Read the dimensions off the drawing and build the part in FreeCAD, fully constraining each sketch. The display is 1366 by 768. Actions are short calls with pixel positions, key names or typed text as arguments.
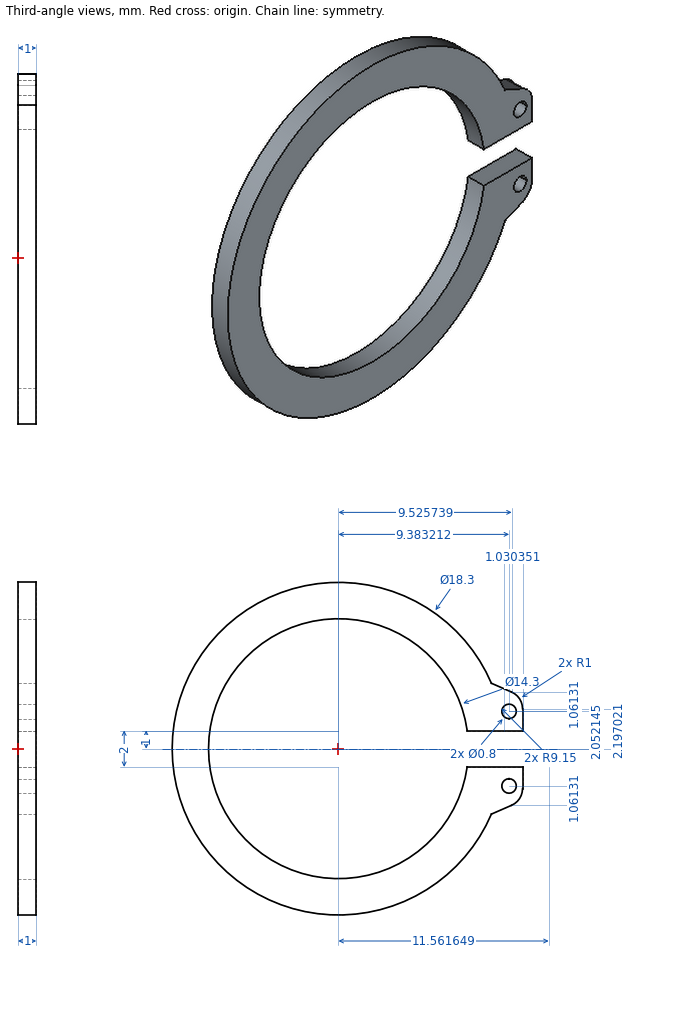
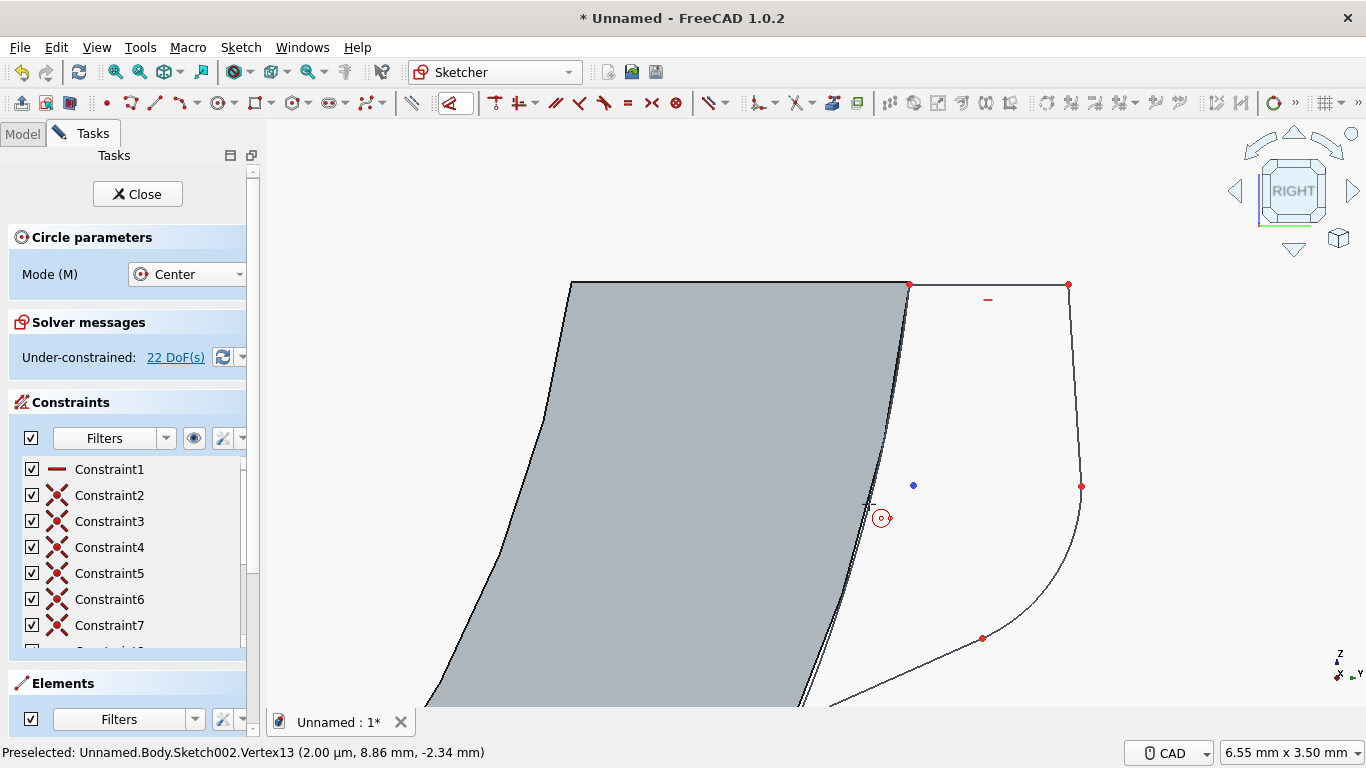
scroll(969, 542, down, 6)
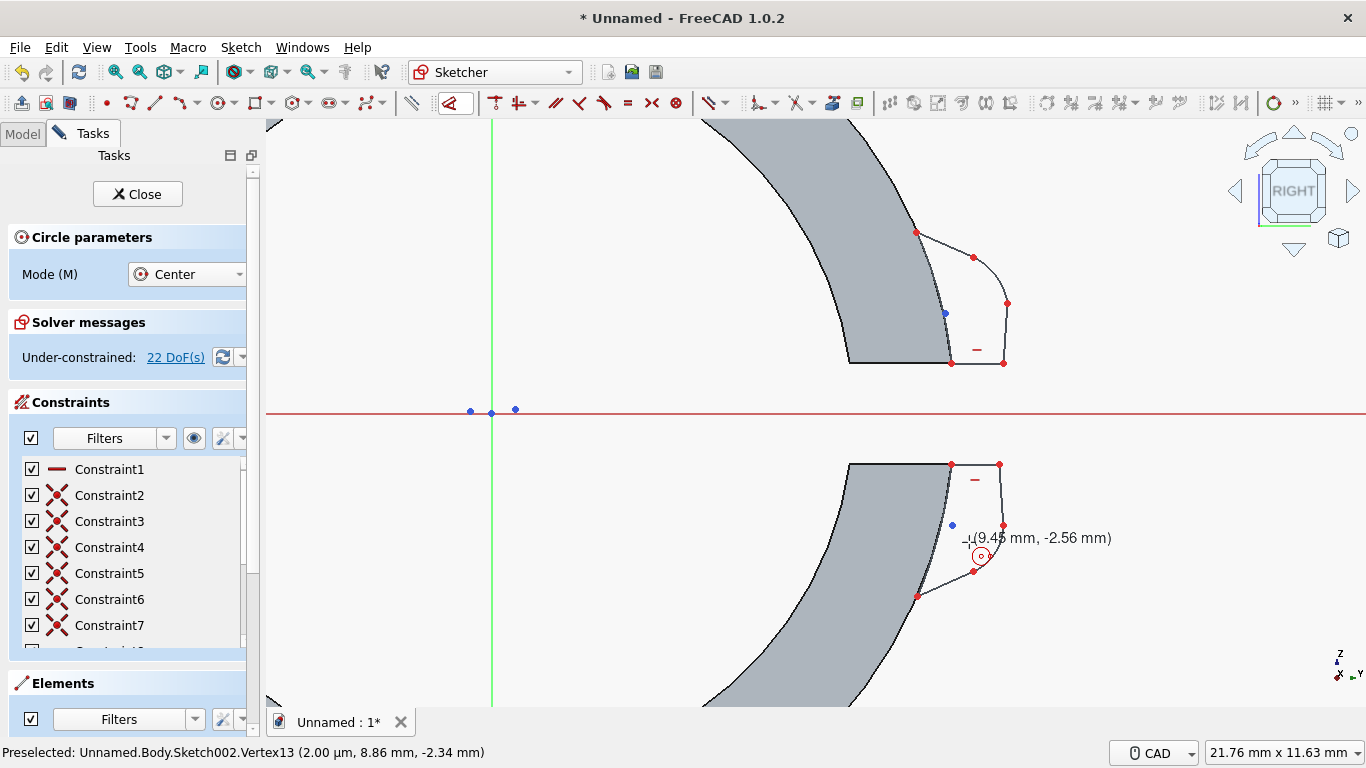
click(966, 310)
click(981, 296)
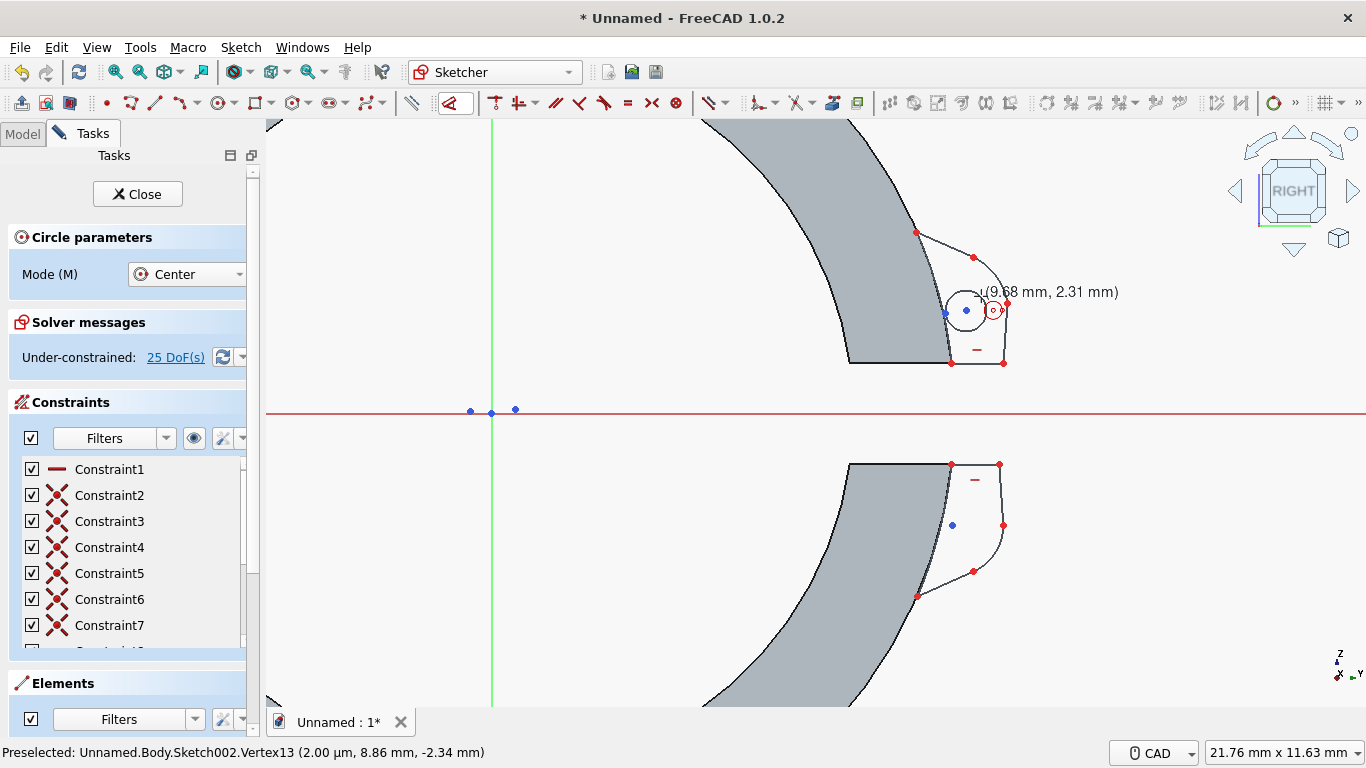
click(966, 517)
click(981, 503)
key(Escape)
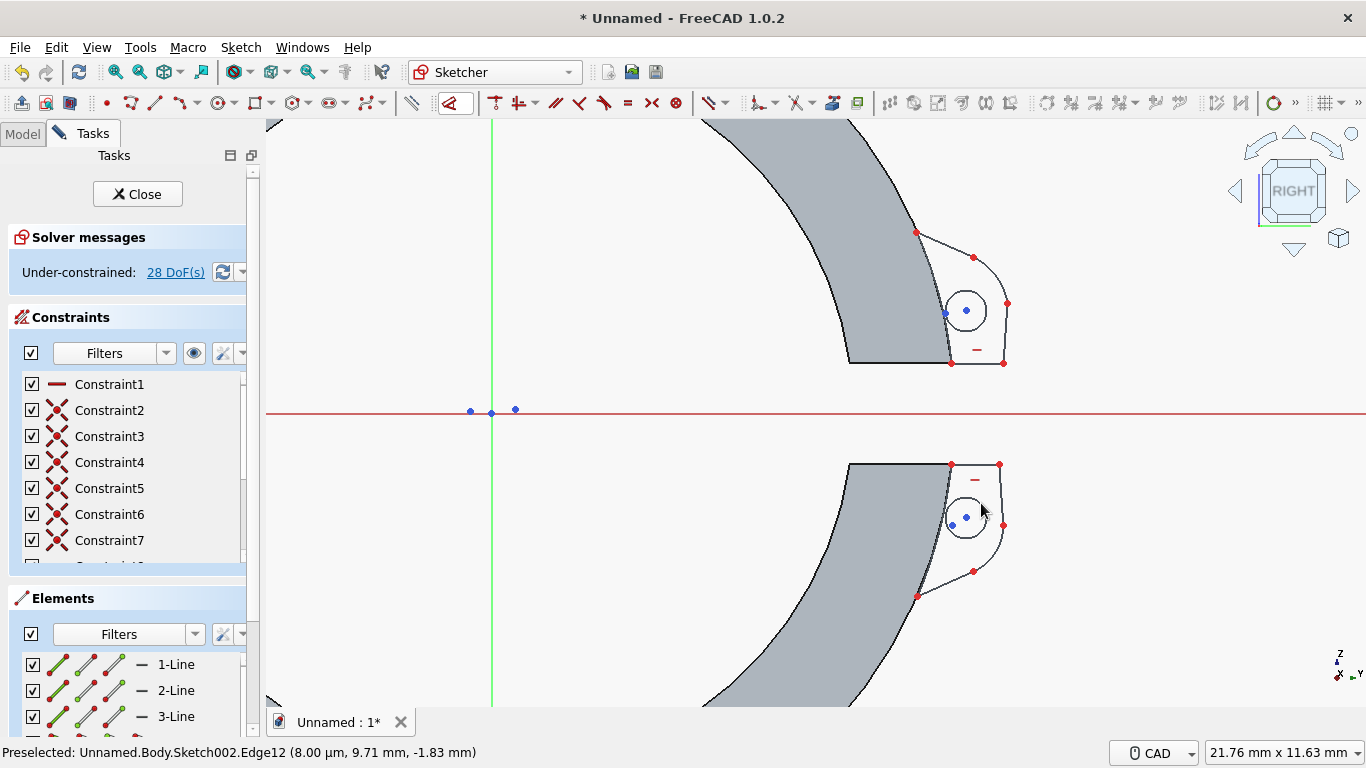
click(1005, 346)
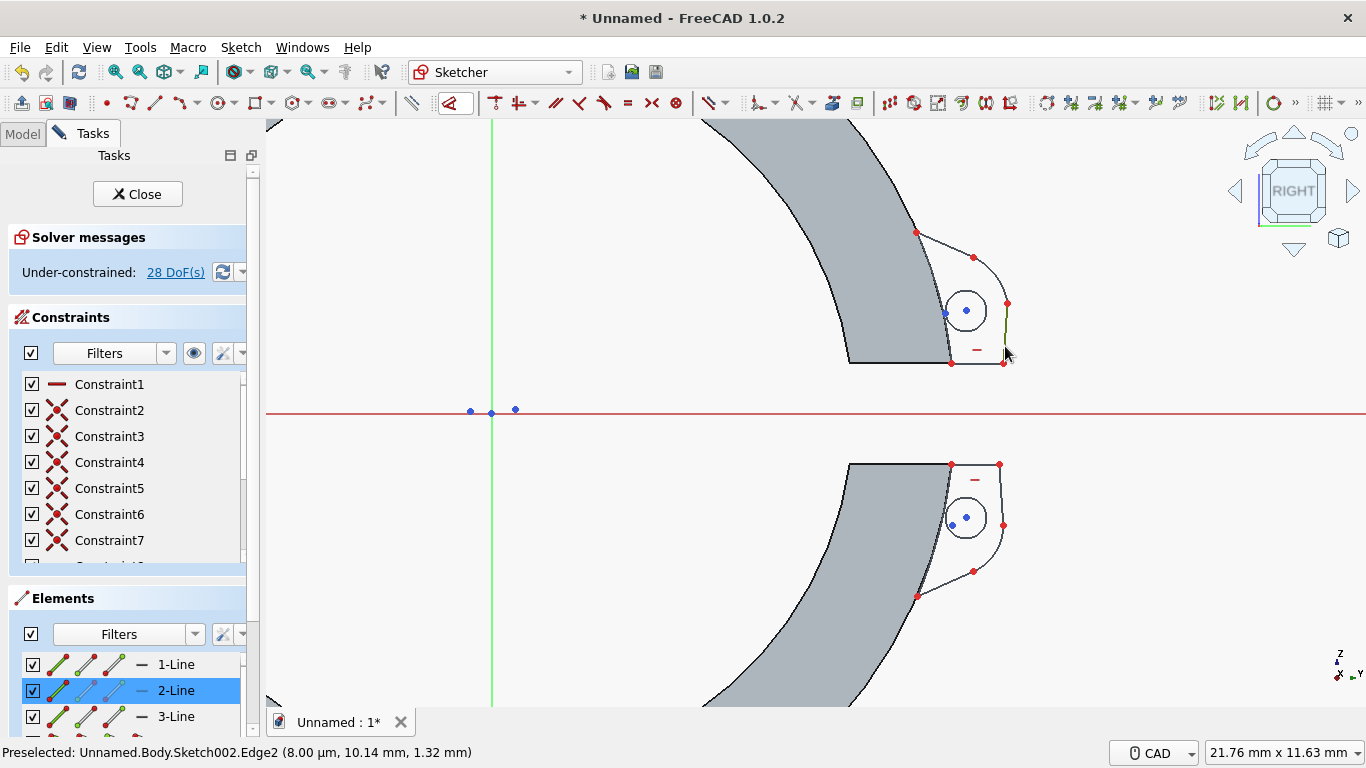
click(1002, 286)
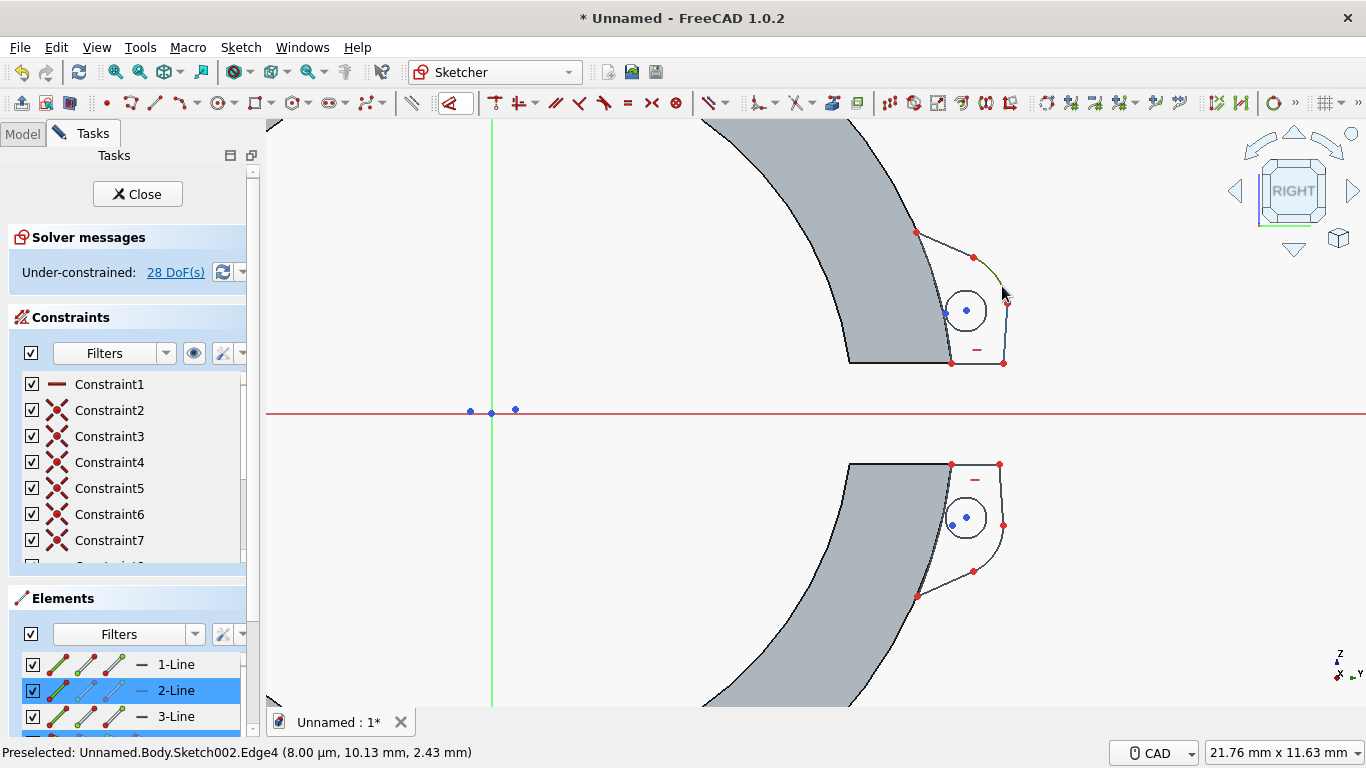
click(604, 104)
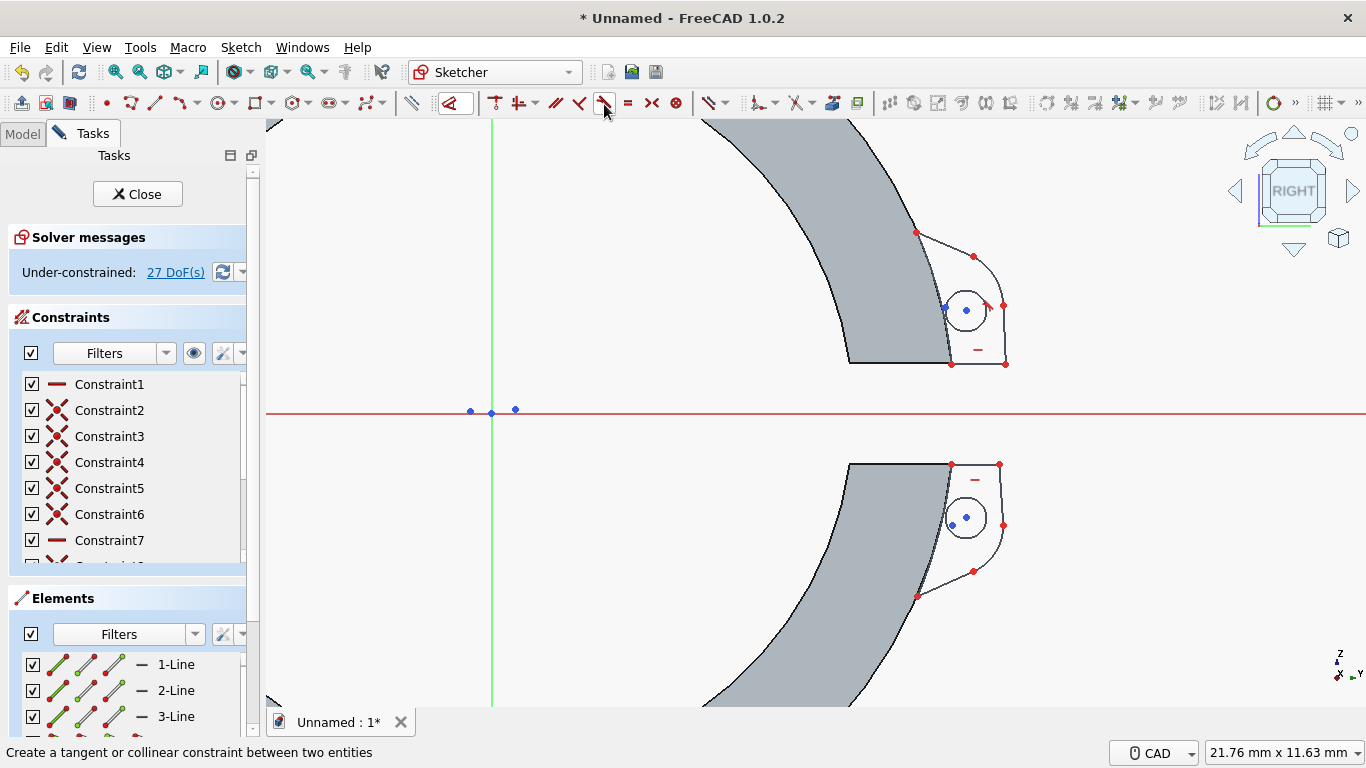
click(957, 249)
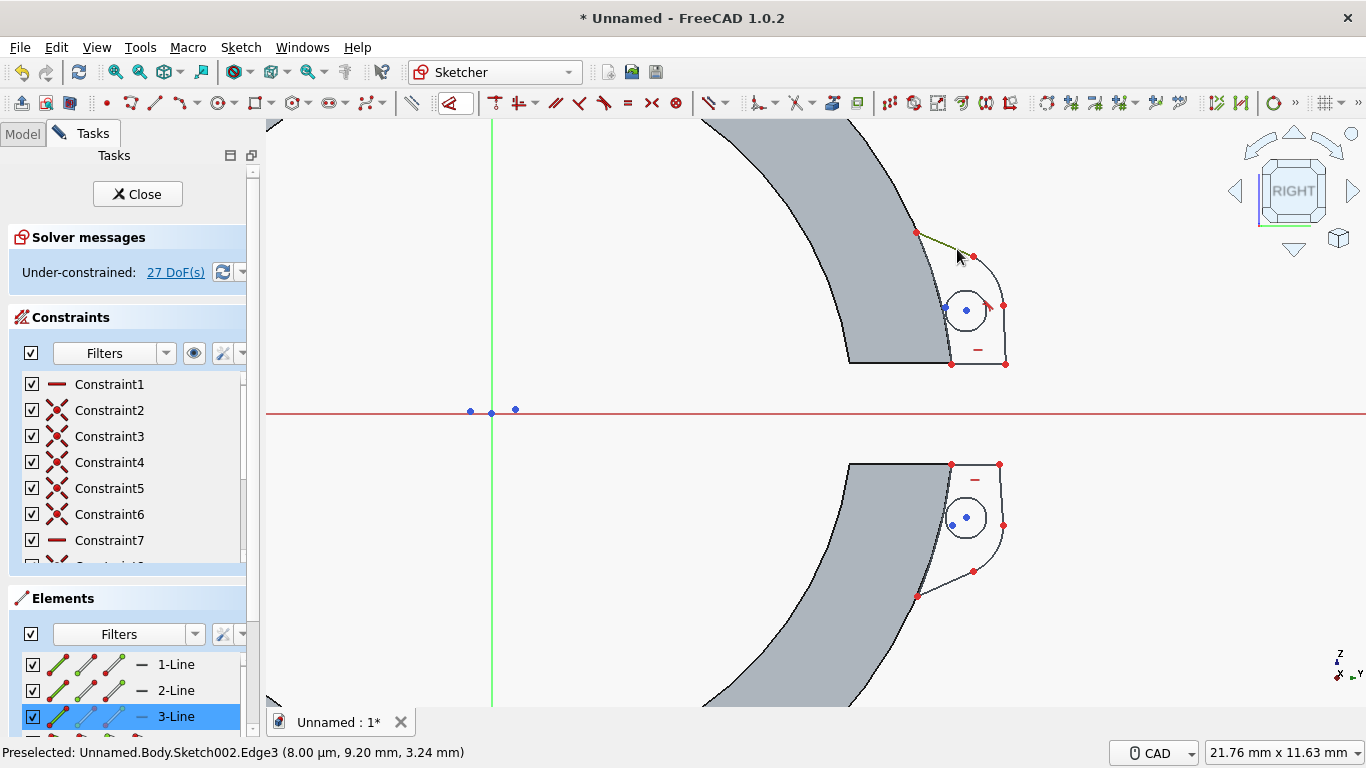
click(1000, 288)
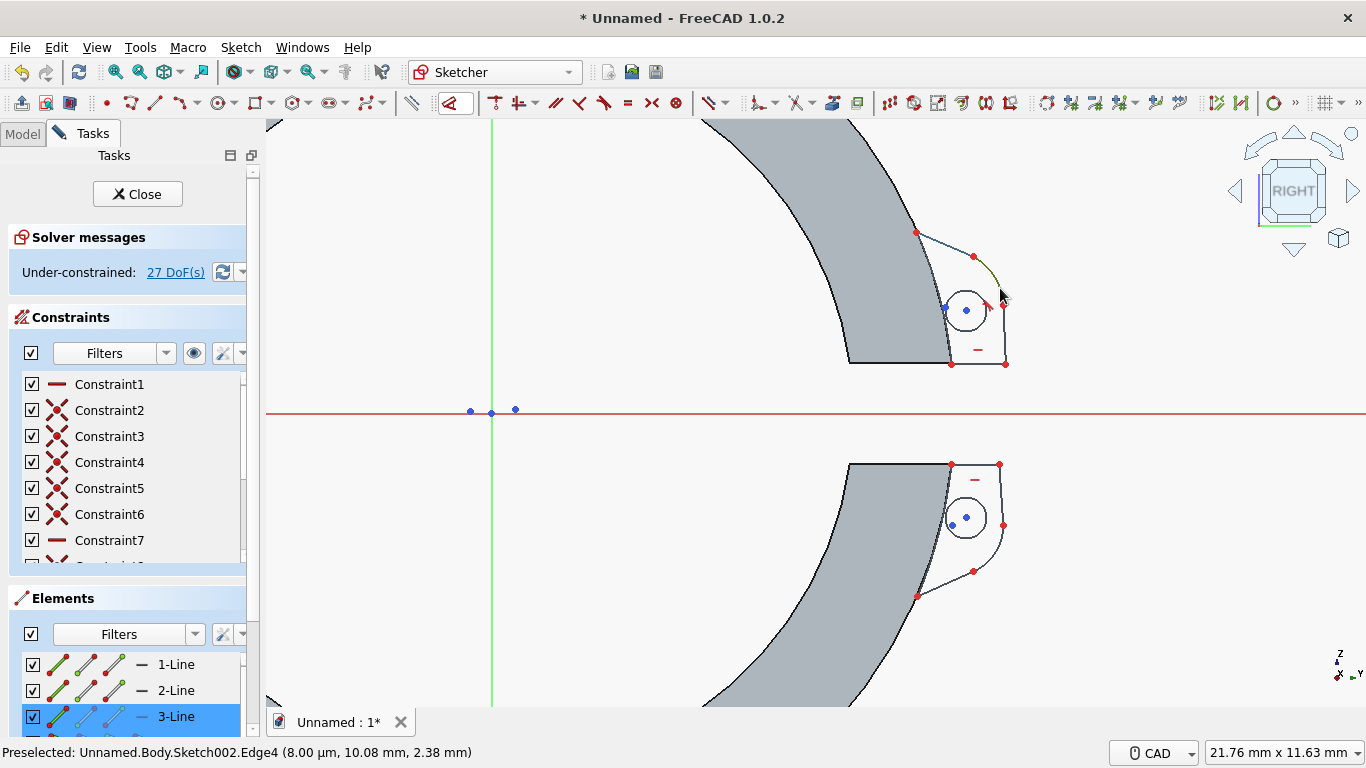
click(604, 104)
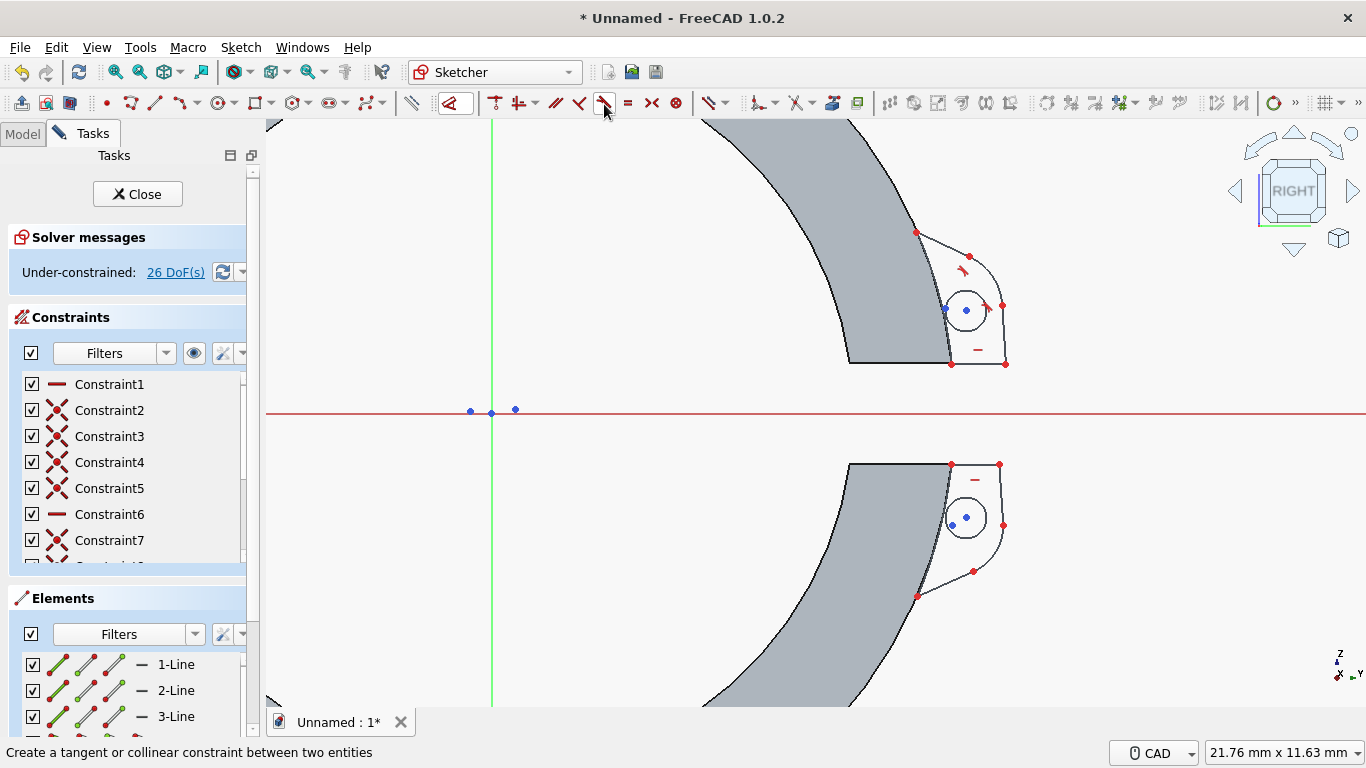
click(934, 589)